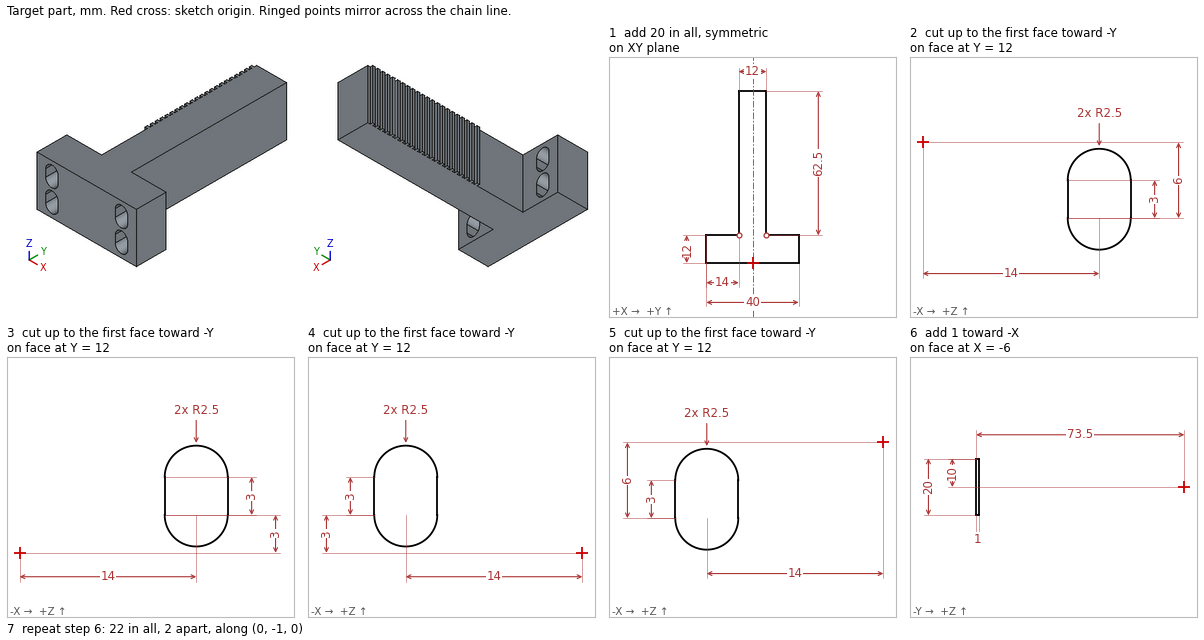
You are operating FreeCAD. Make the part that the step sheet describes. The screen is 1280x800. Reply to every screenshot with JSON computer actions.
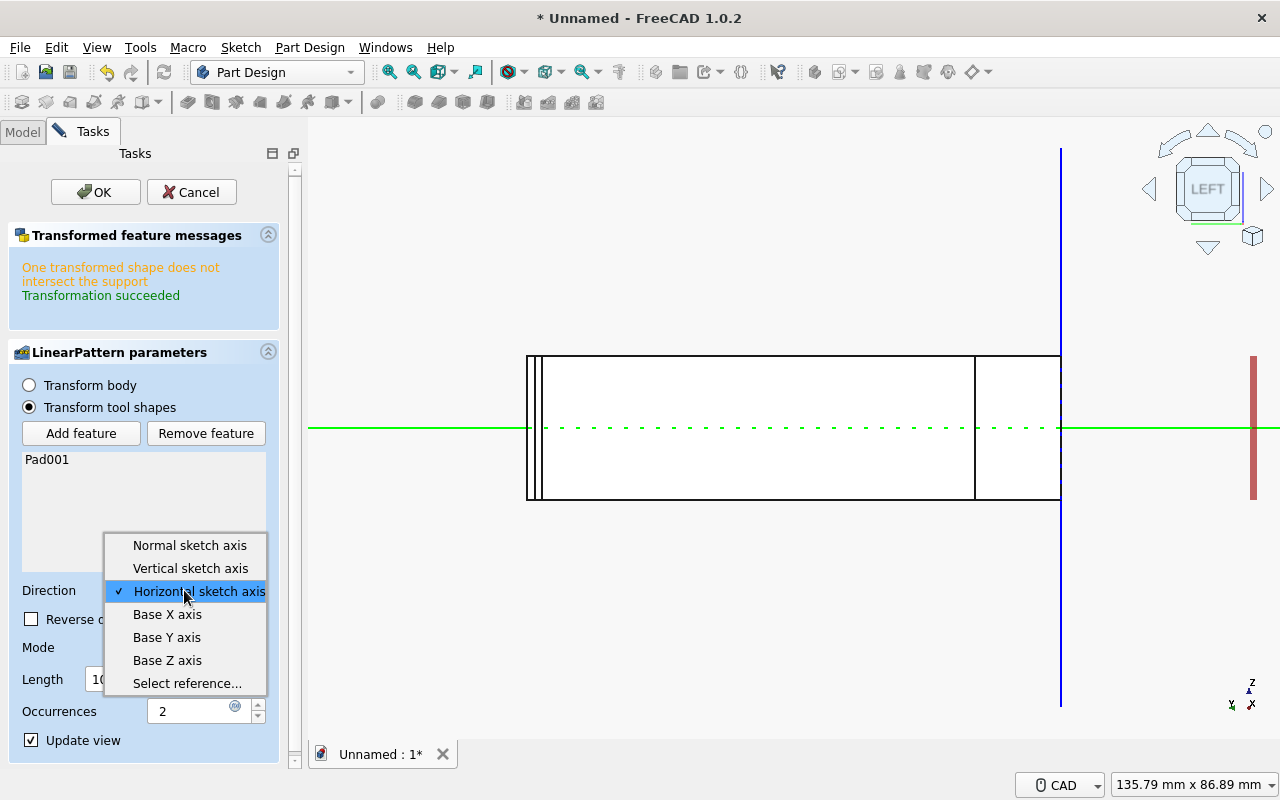
{"action": "left_click", "coordinate": [184, 638]}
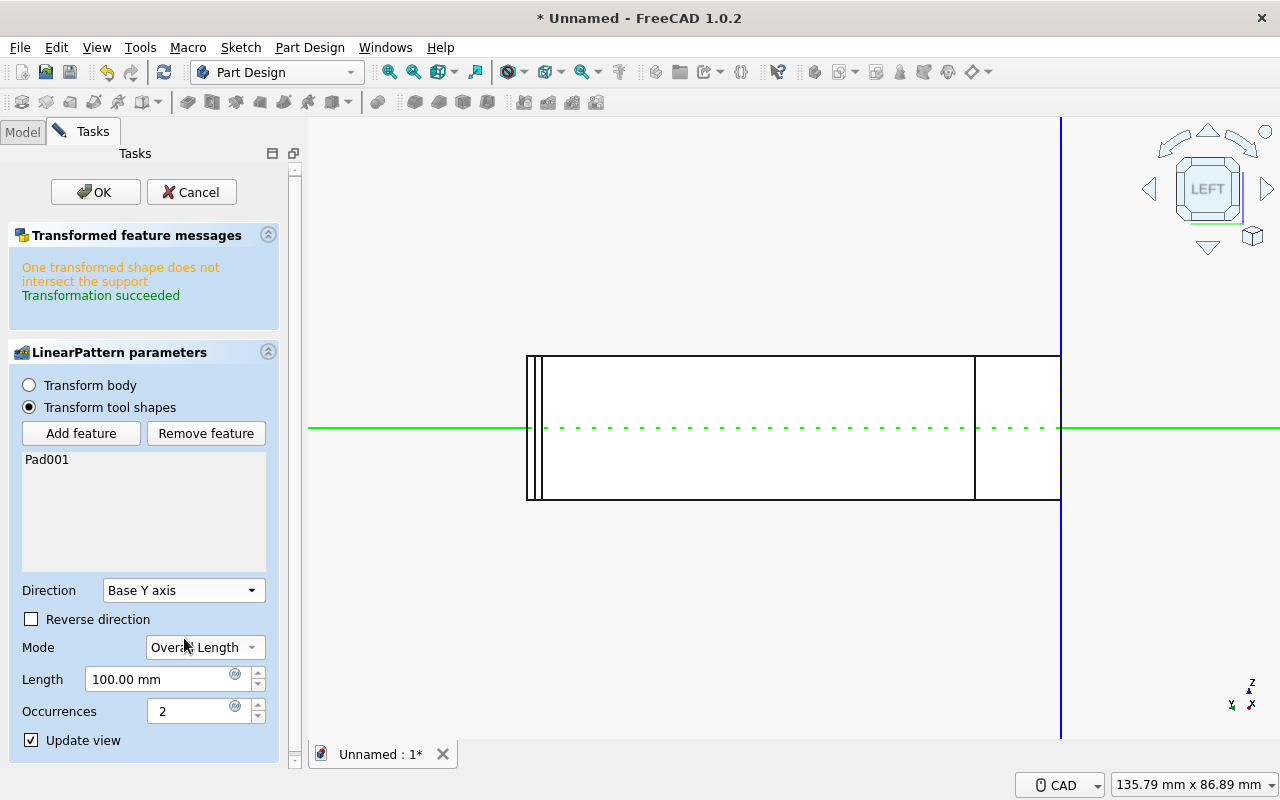
{"action": "left_click", "coordinate": [206, 648]}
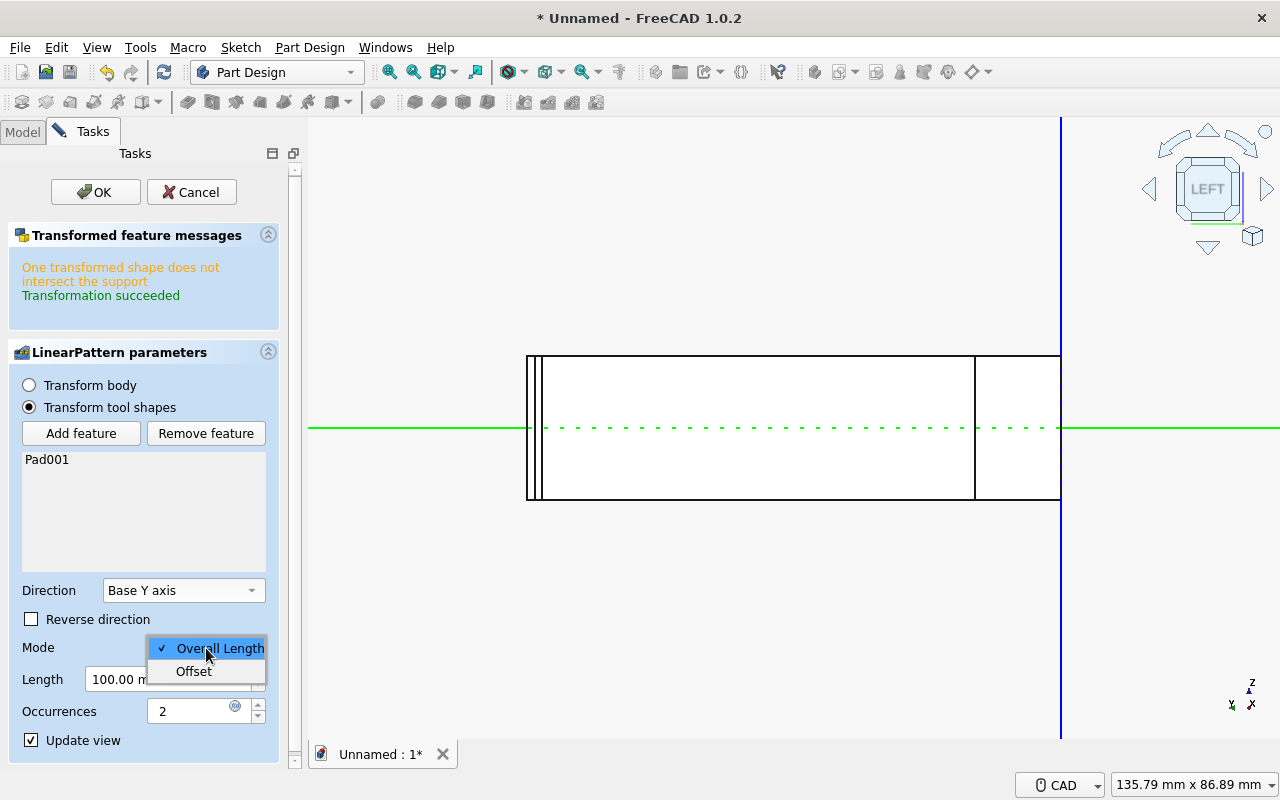
{"action": "left_click", "coordinate": [206, 672]}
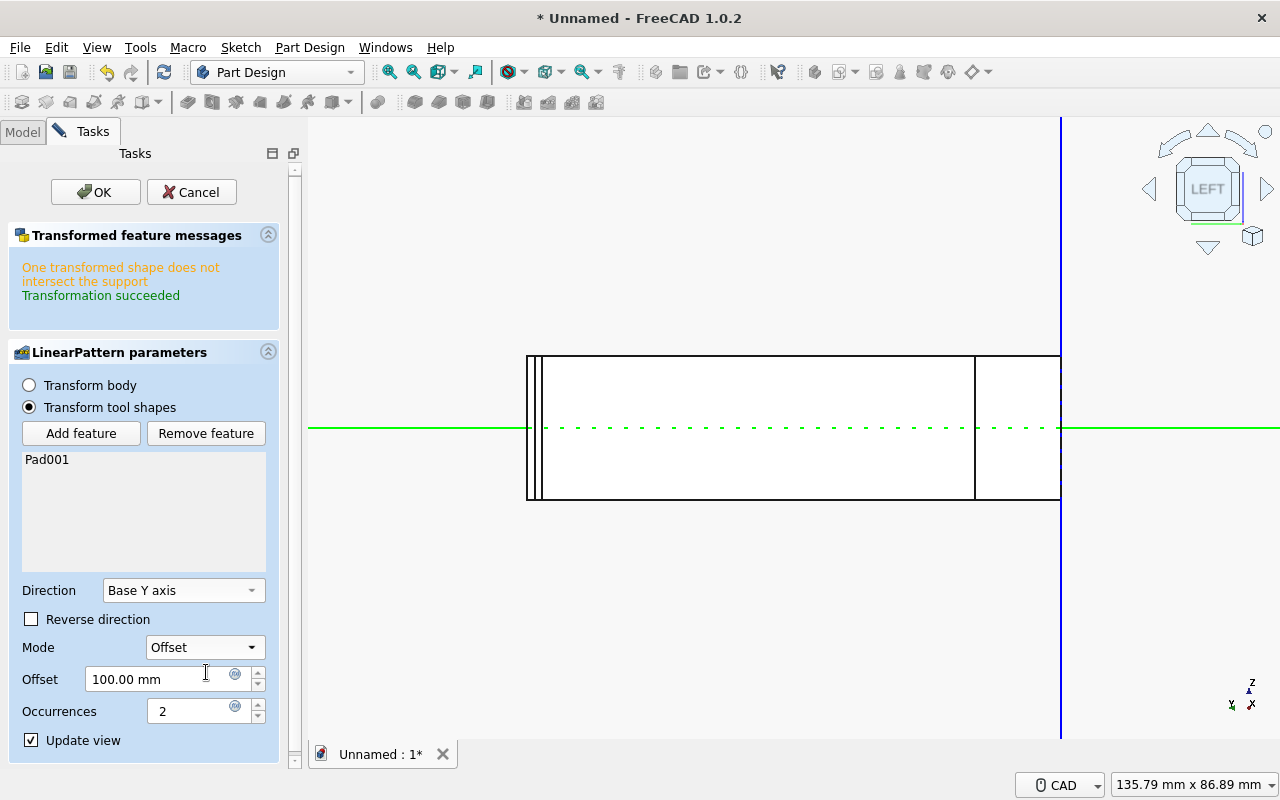
{"action": "triple_click", "coordinate": [168, 679]}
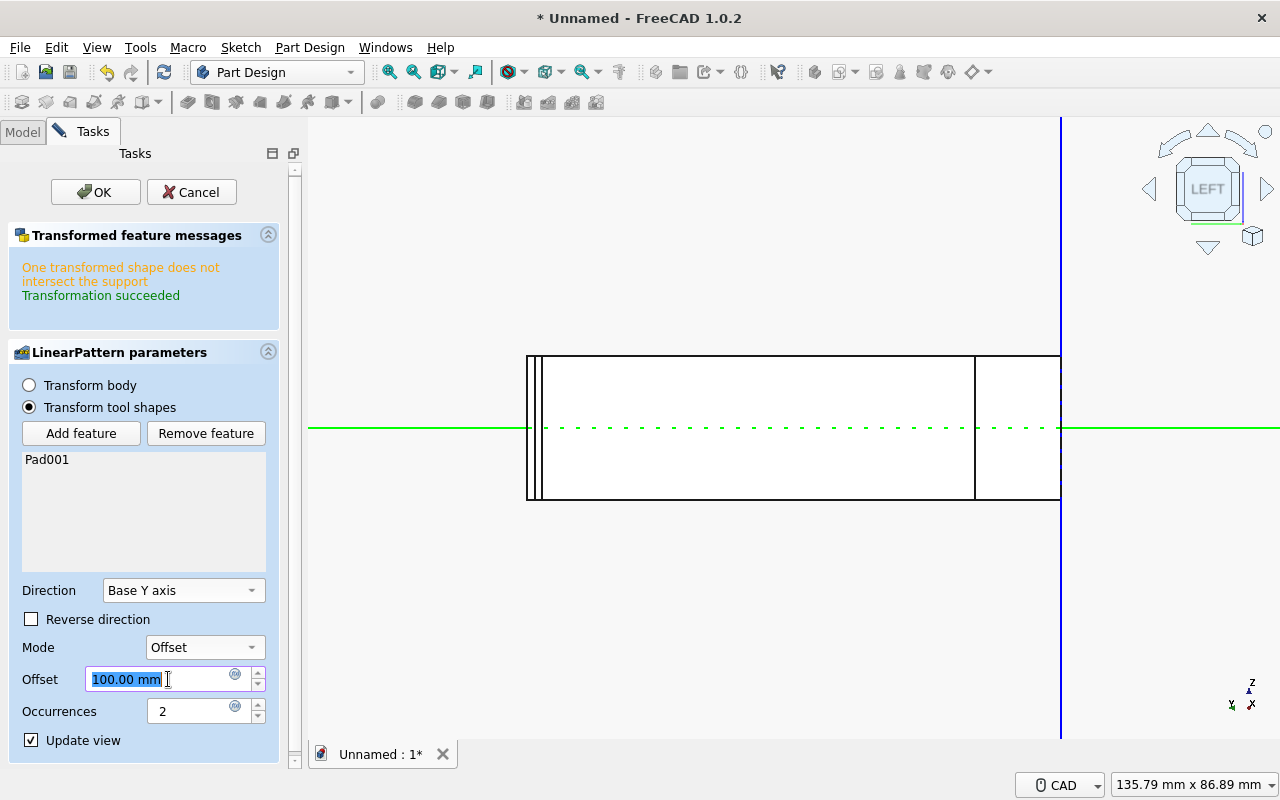
{"action": "type", "text": "2"}
{"action": "key", "text": "Tab"}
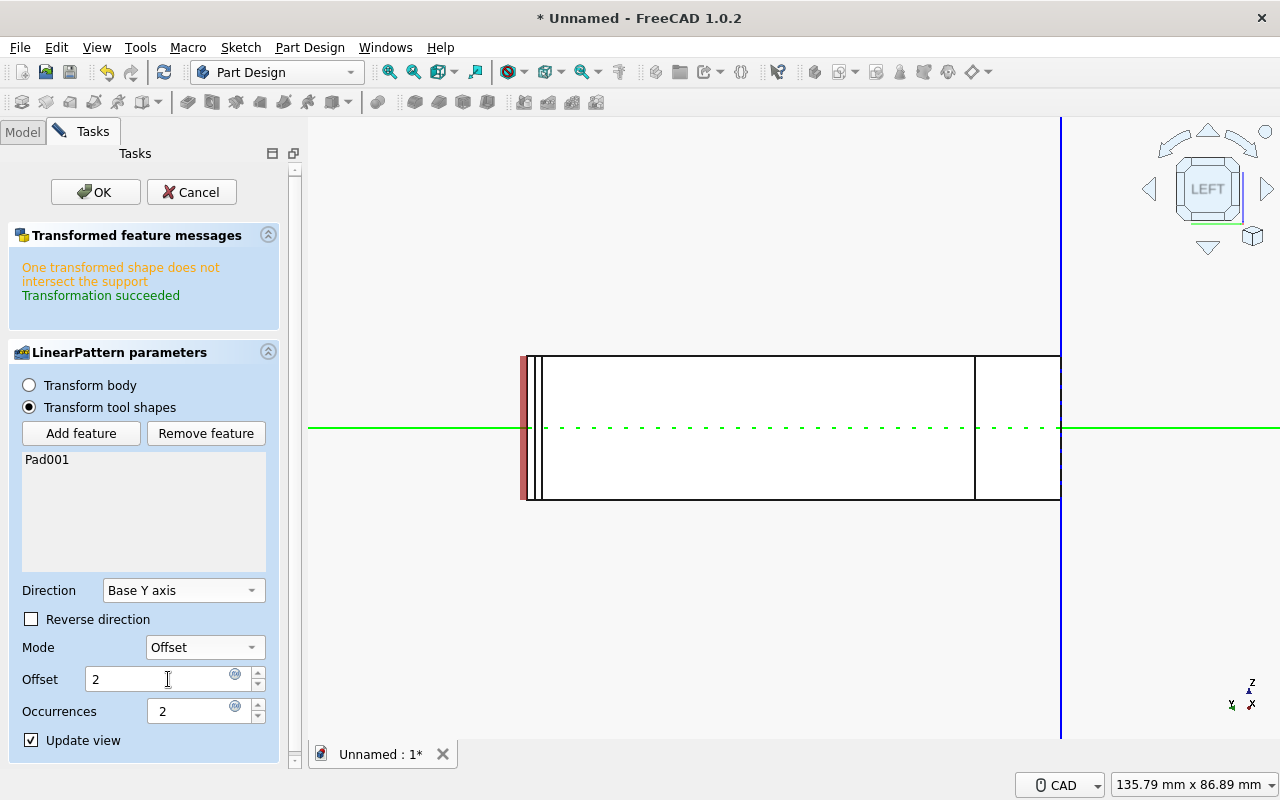
{"action": "triple_click", "coordinate": [198, 711]}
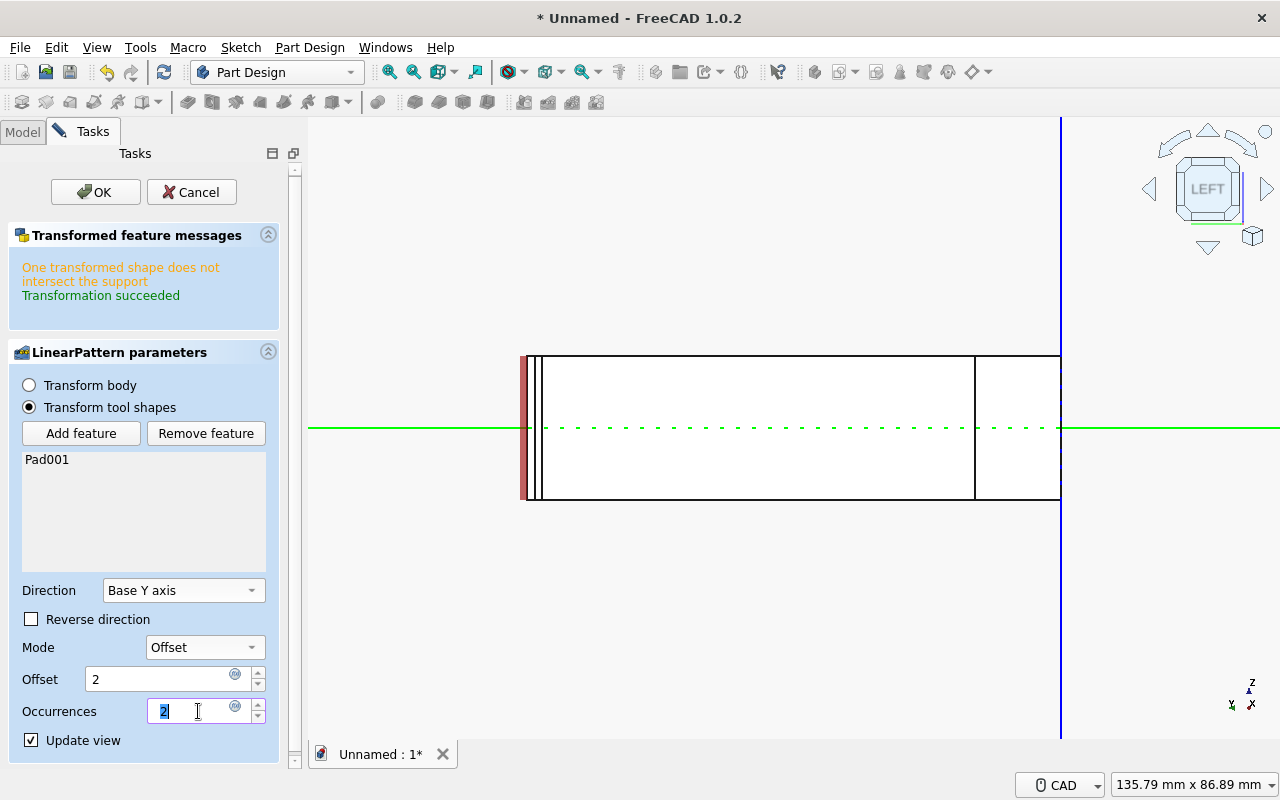
{"action": "type", "text": "22"}
{"action": "key", "text": "Tab"}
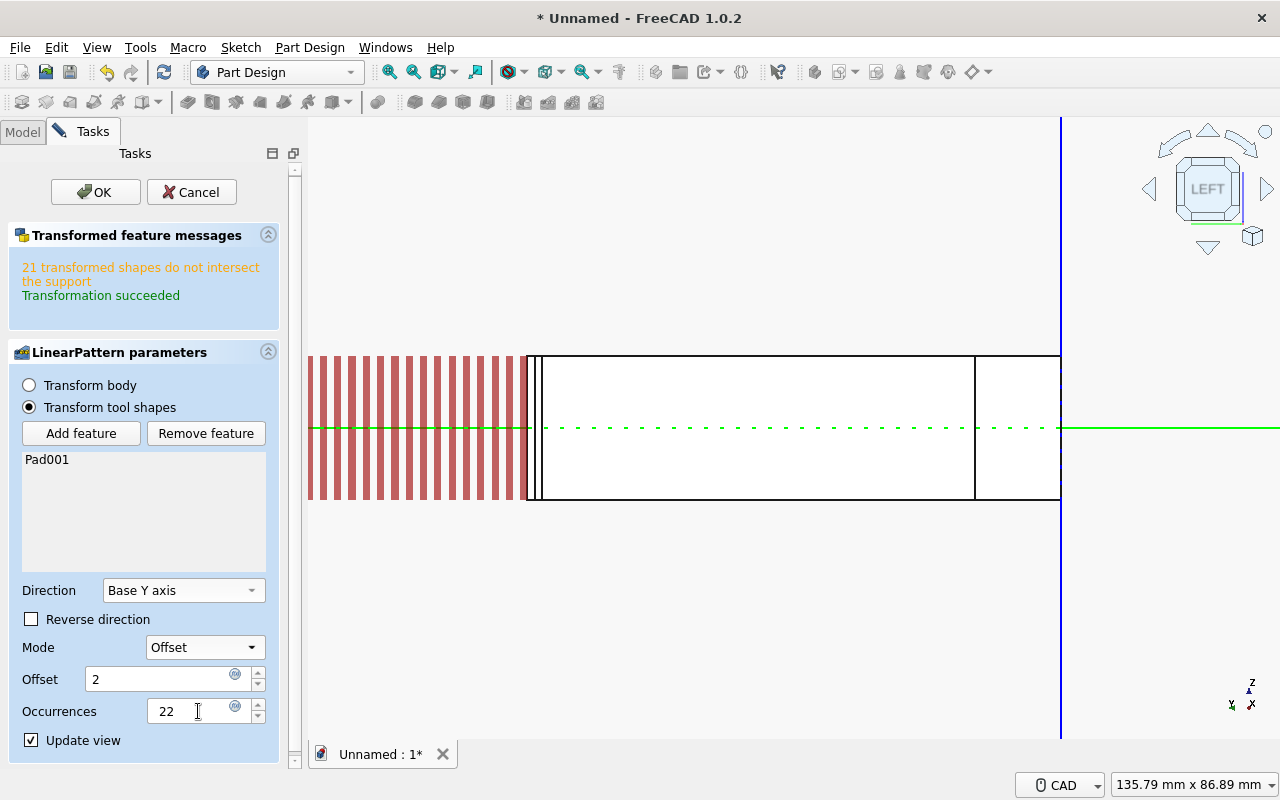
{"action": "left_click", "coordinate": [30, 619]}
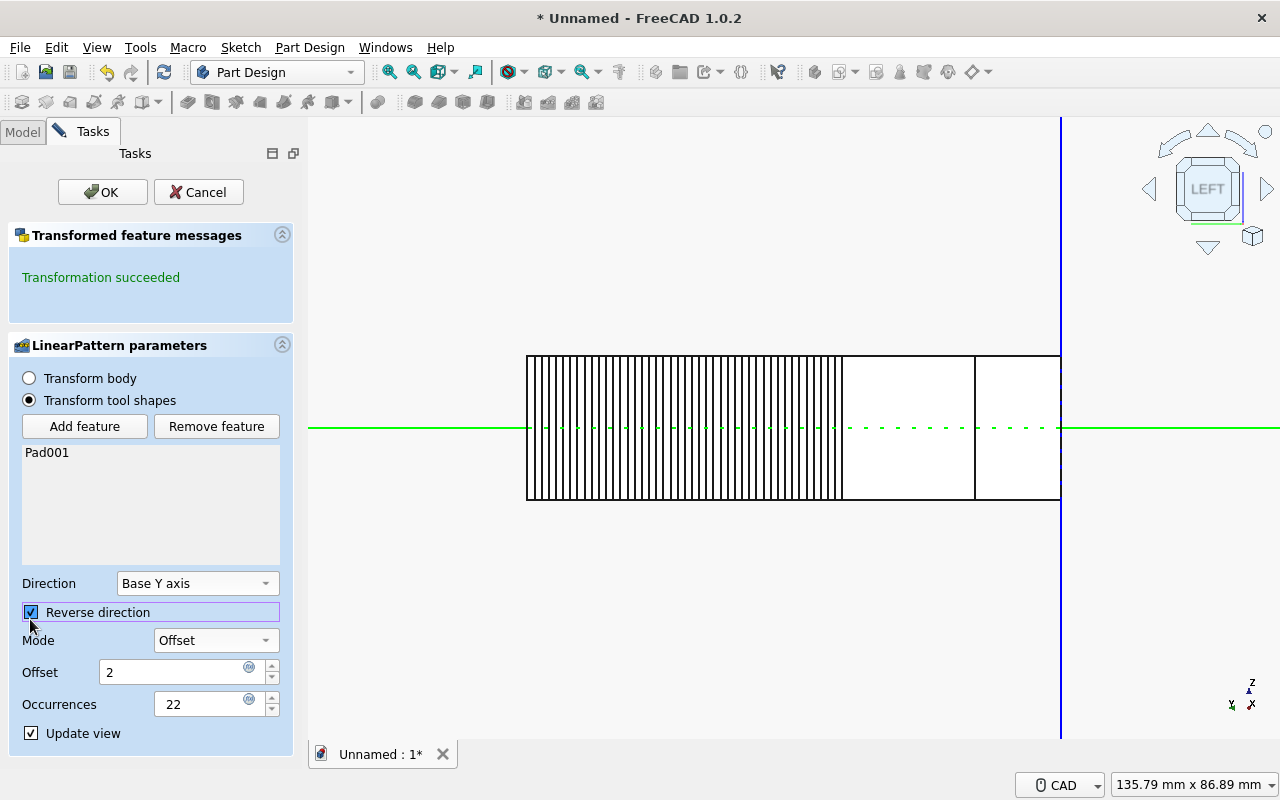
{"action": "left_click", "coordinate": [103, 192]}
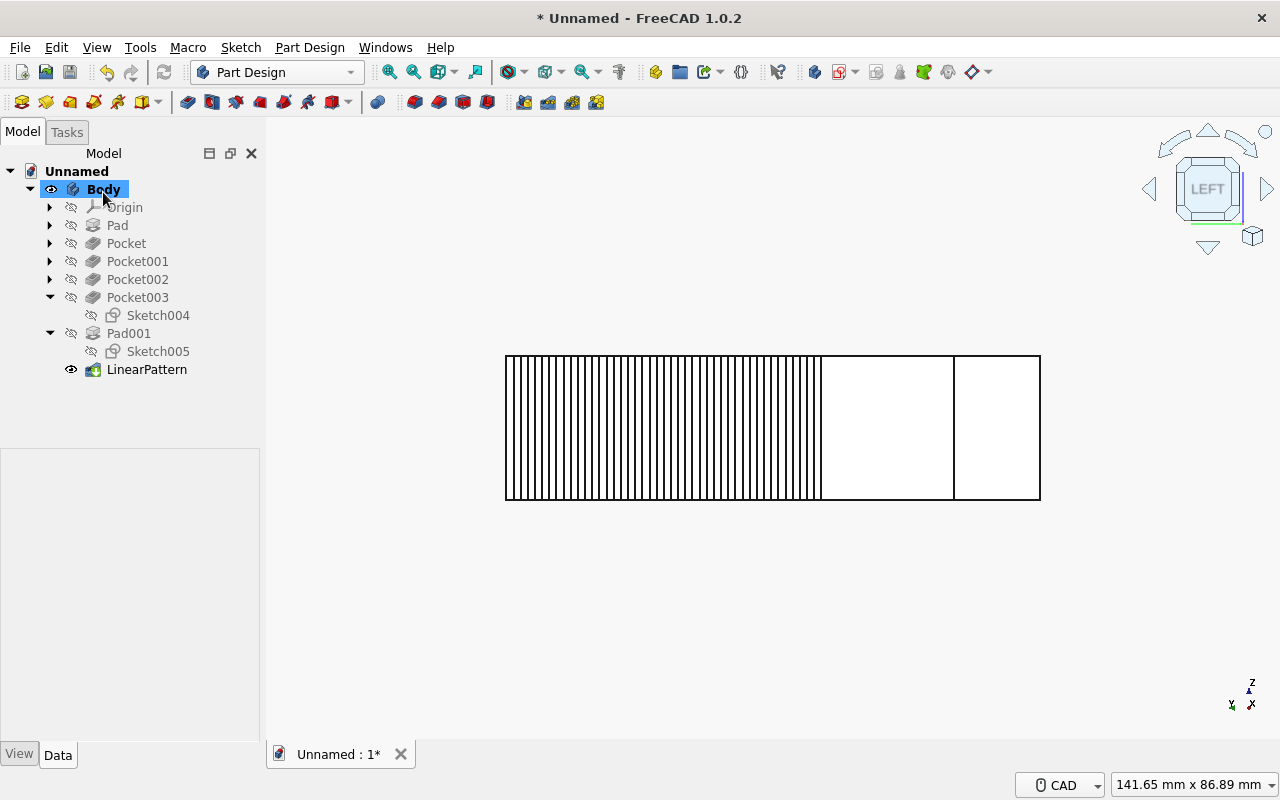
{"action": "key", "text": "0"}